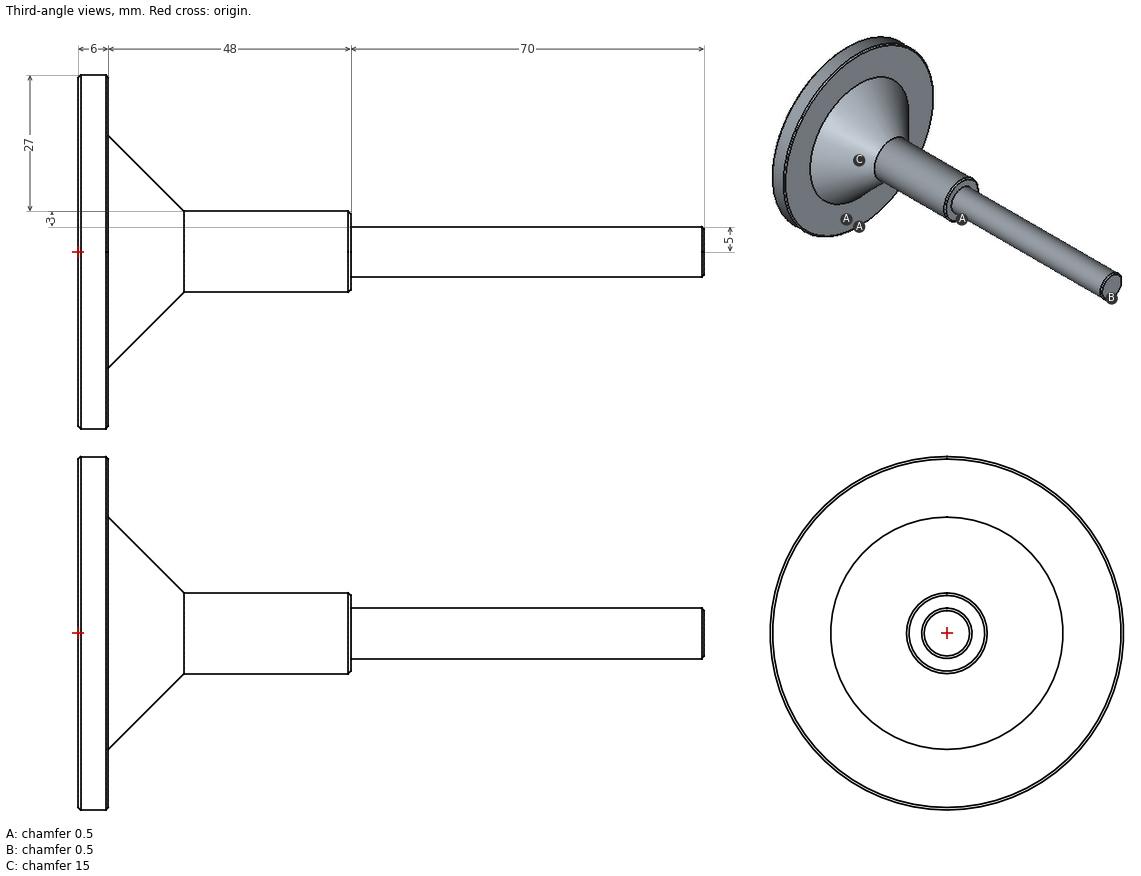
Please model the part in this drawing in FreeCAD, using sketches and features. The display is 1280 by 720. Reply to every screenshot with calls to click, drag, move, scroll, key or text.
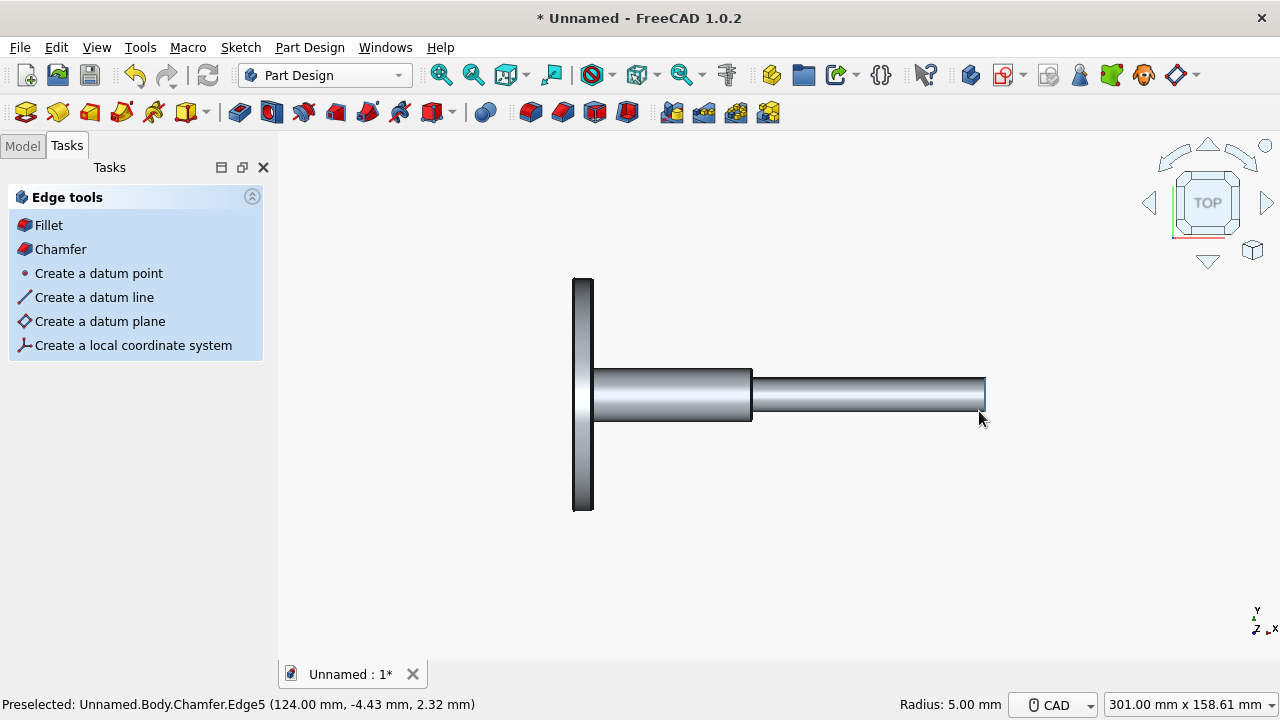
click(564, 112)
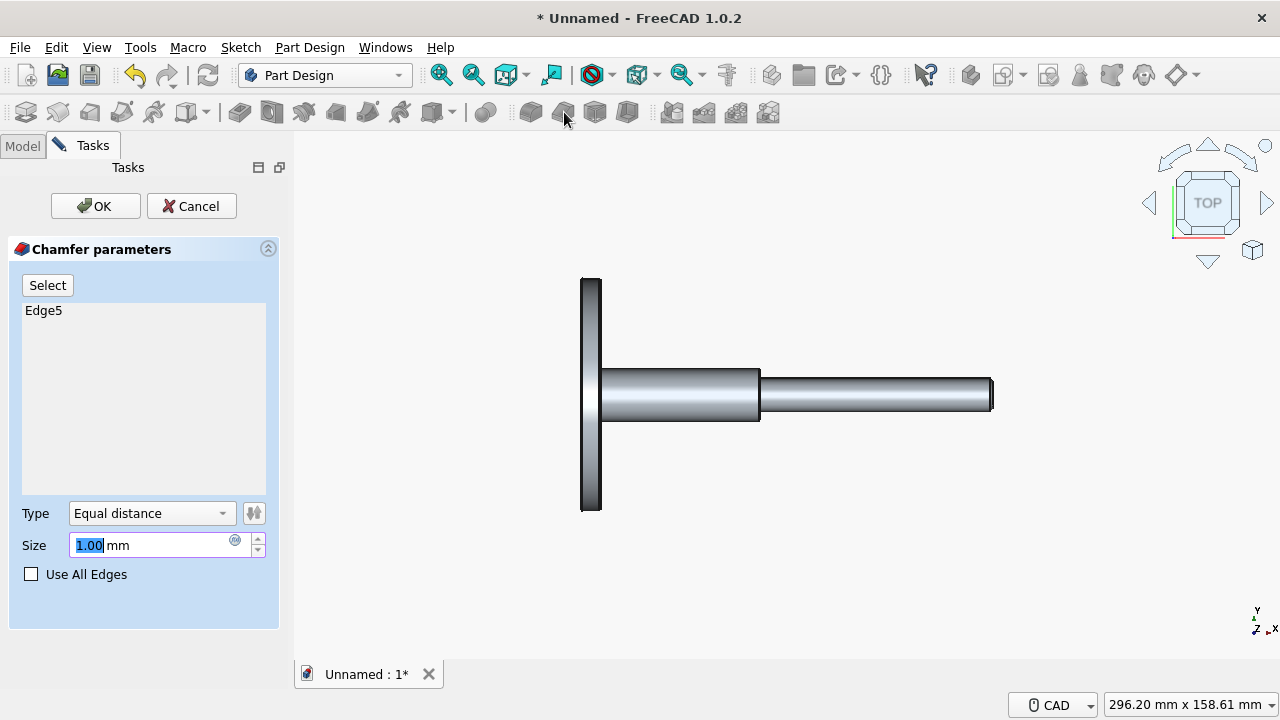
text(0.5)
key(Tab)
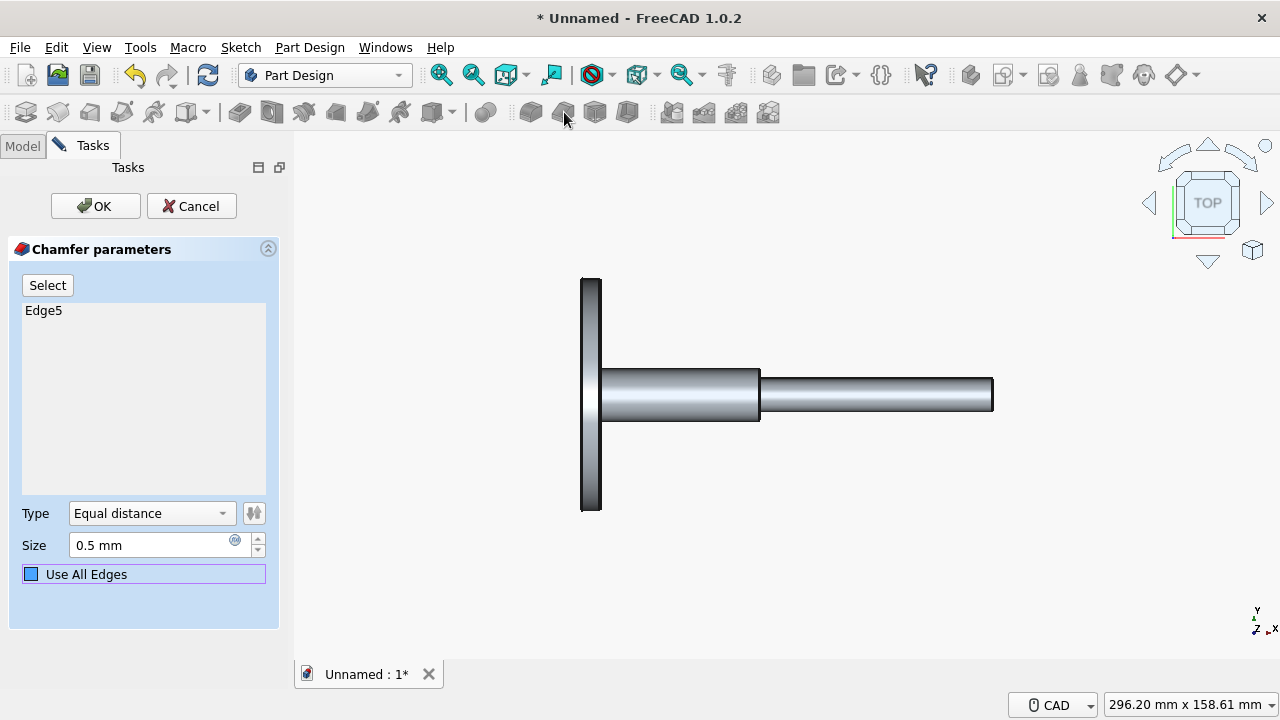
click(96, 206)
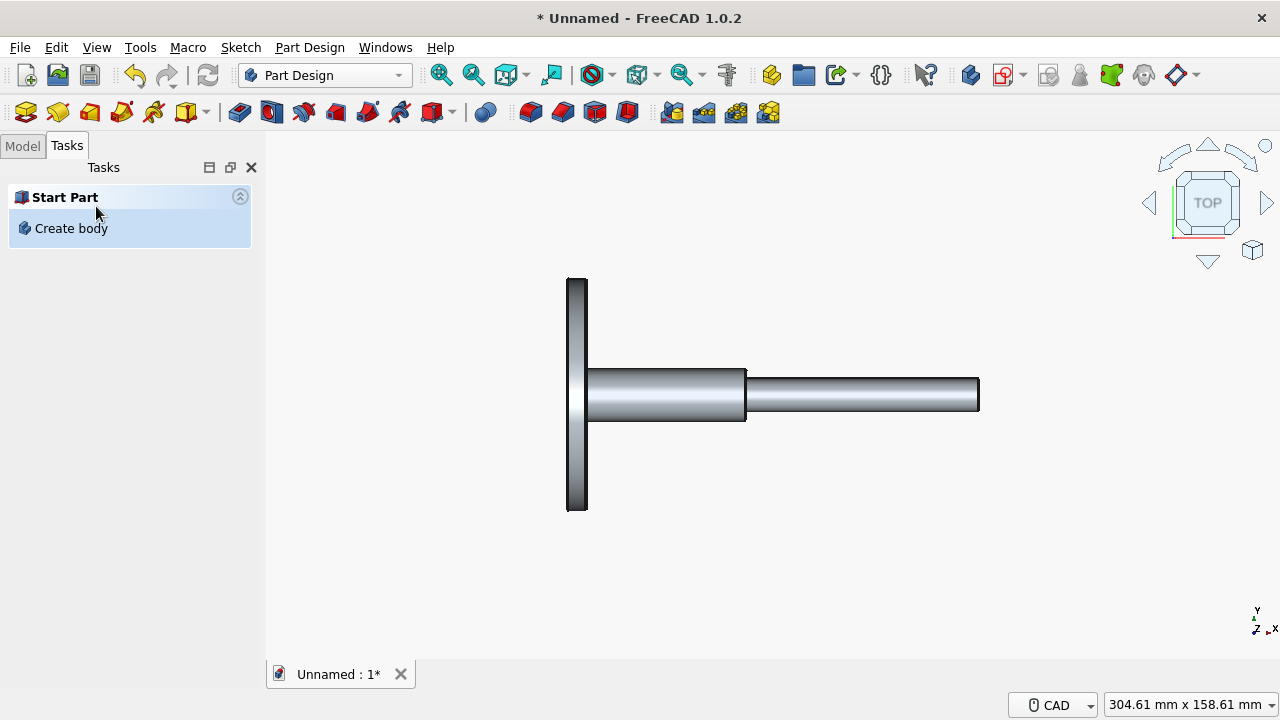
click(442, 76)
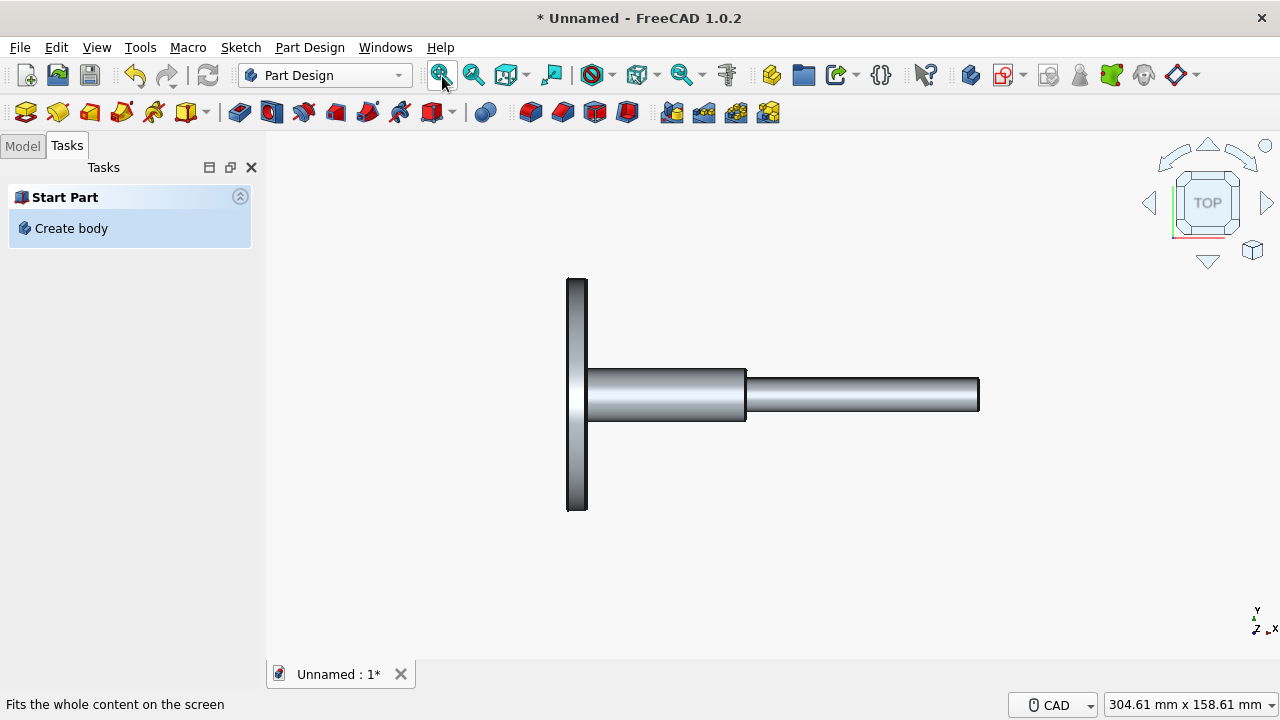
key(0)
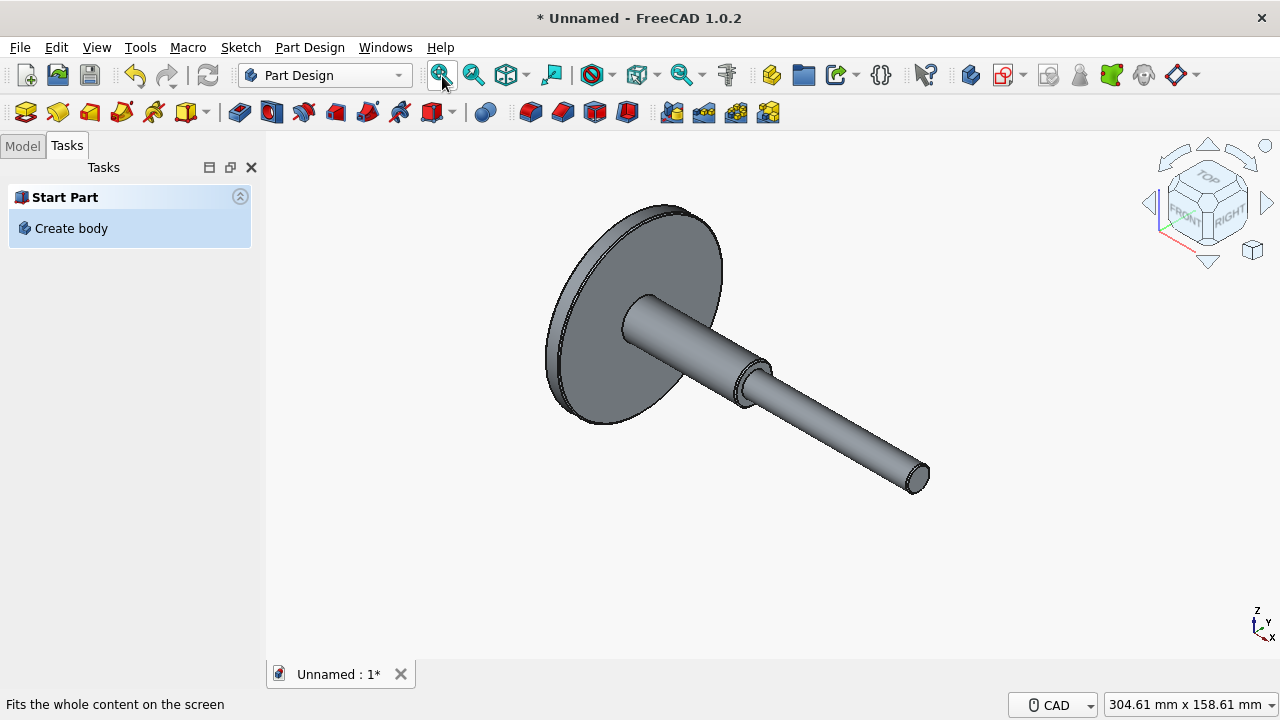
key(2)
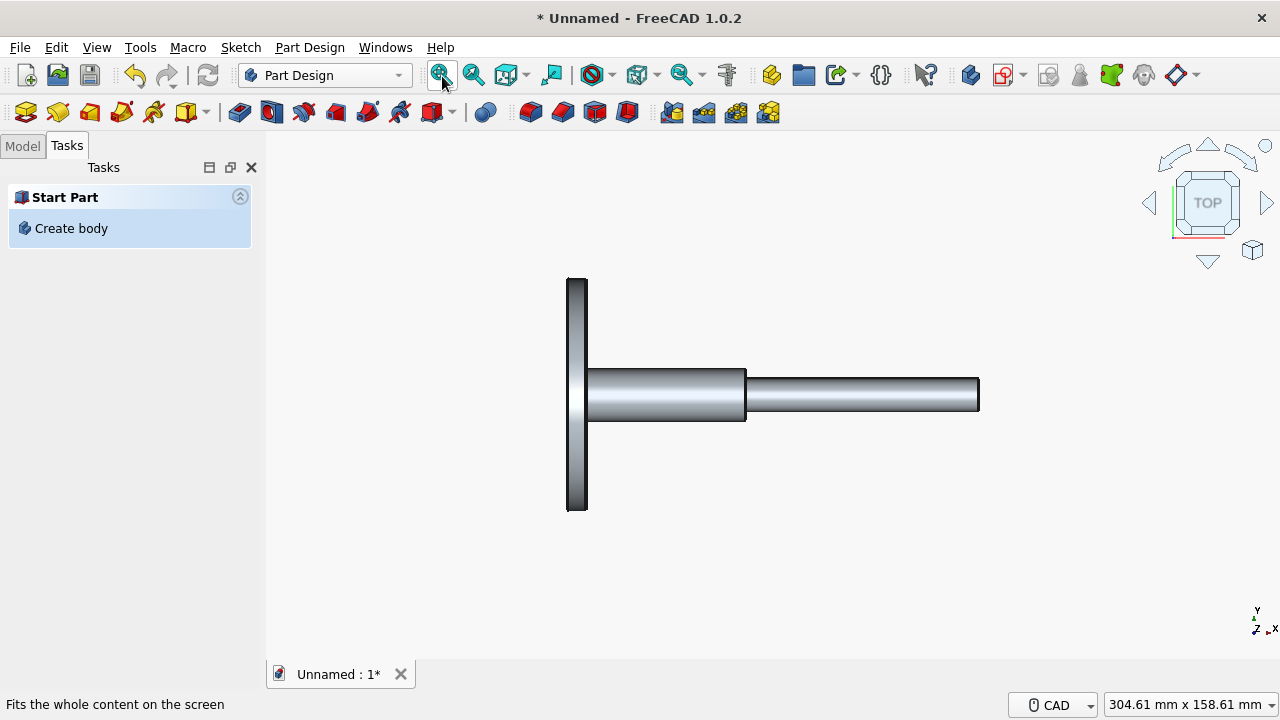
click(442, 76)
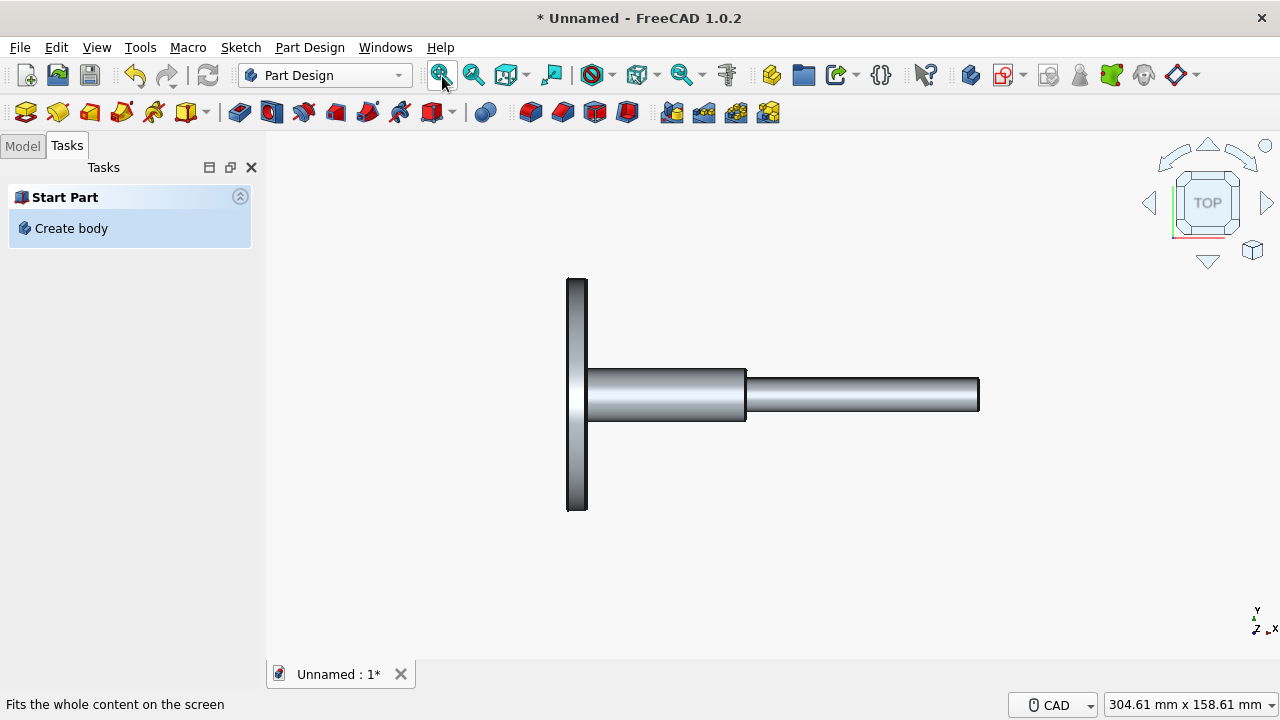
key(1)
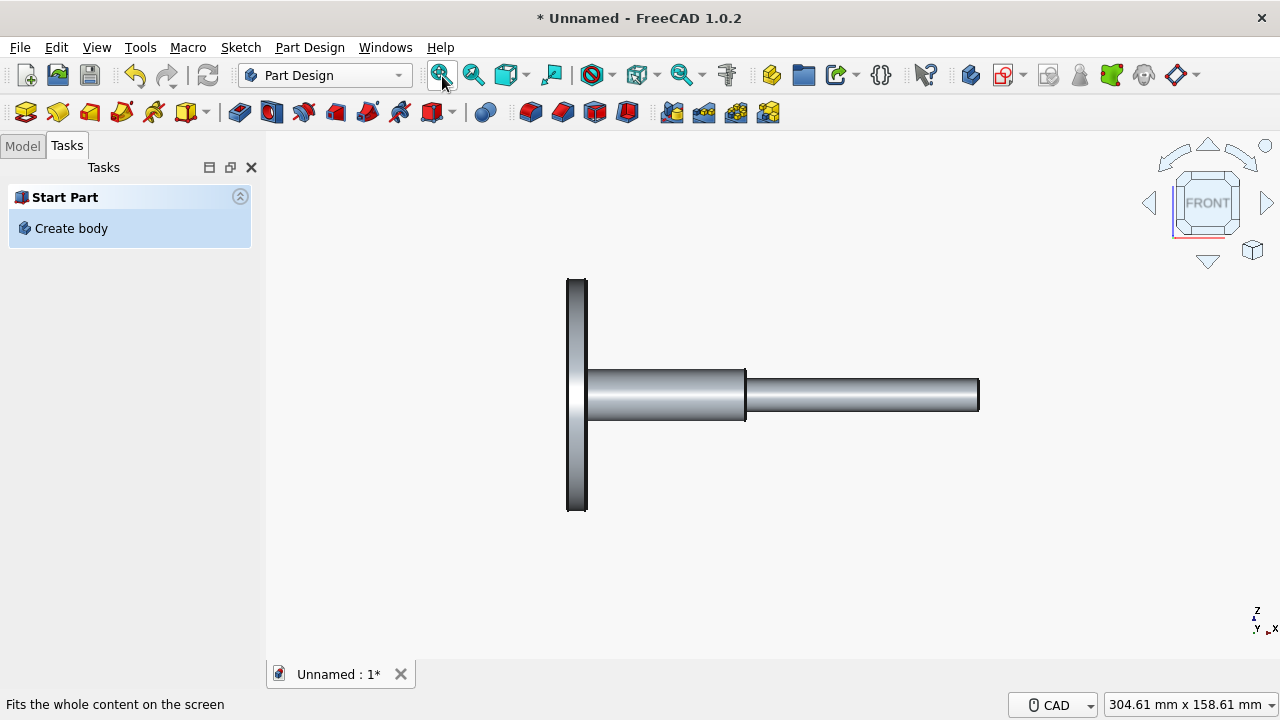
click(442, 76)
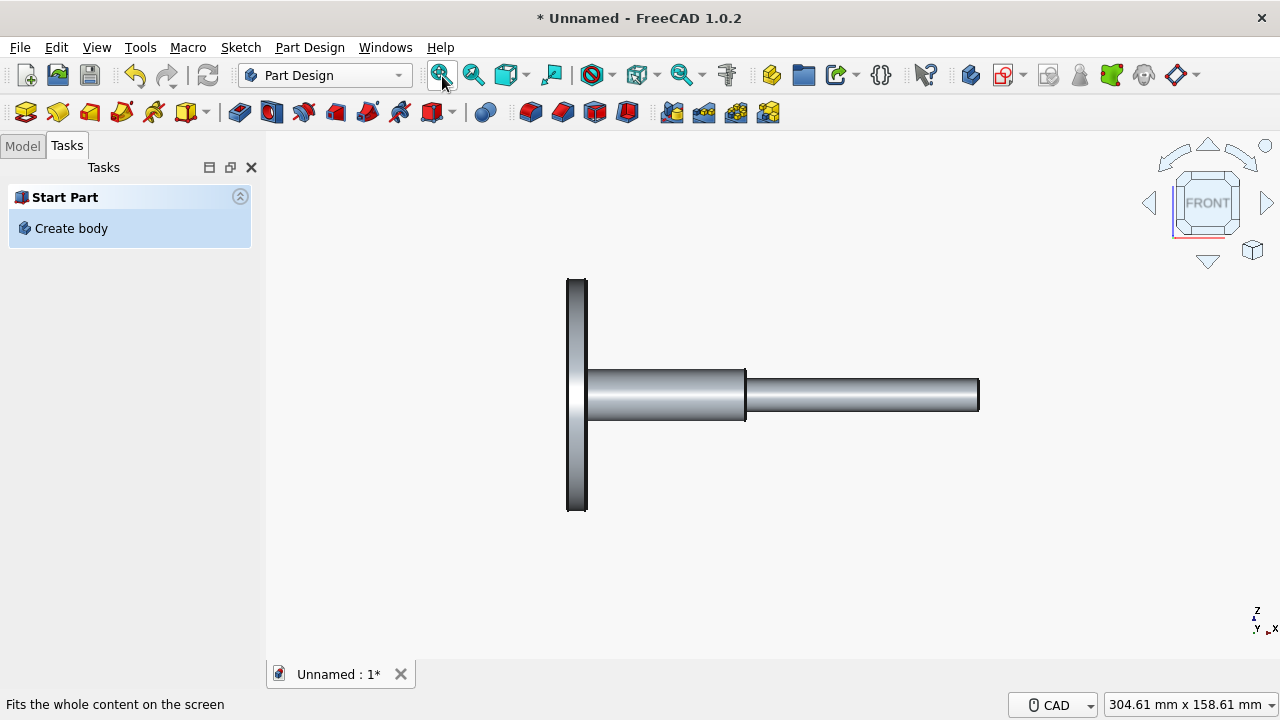
key(3)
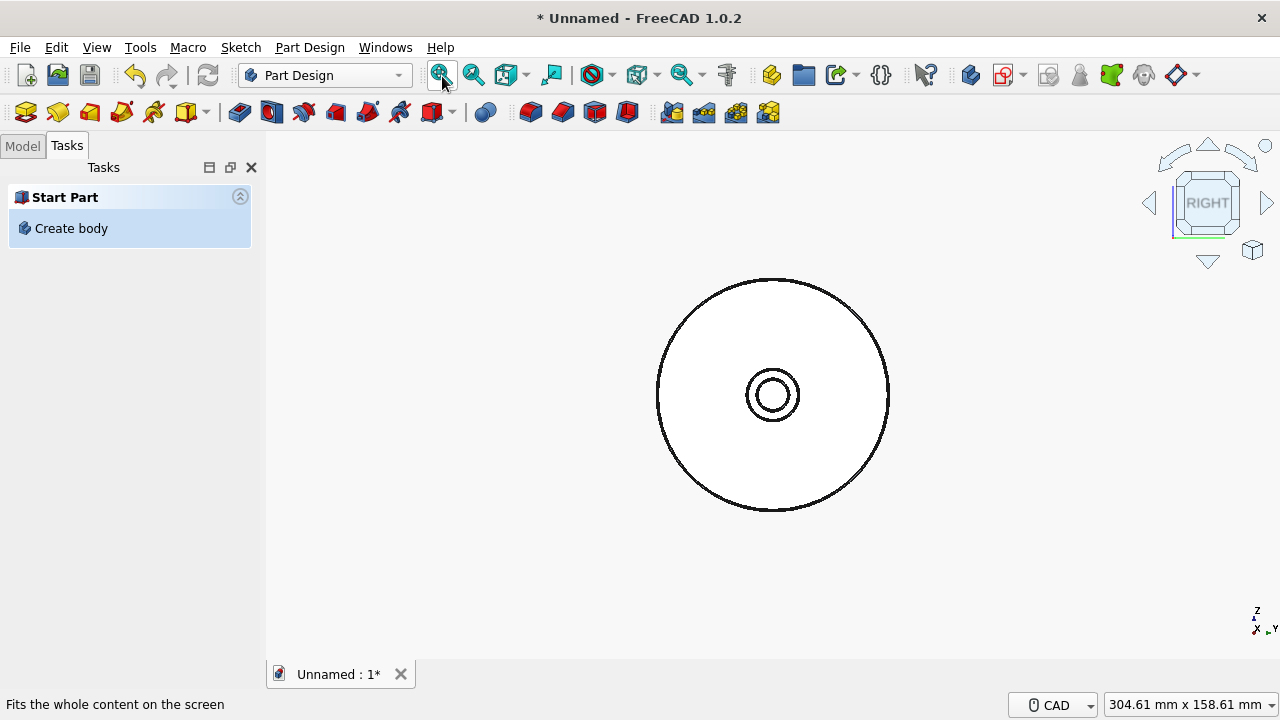
click(442, 76)